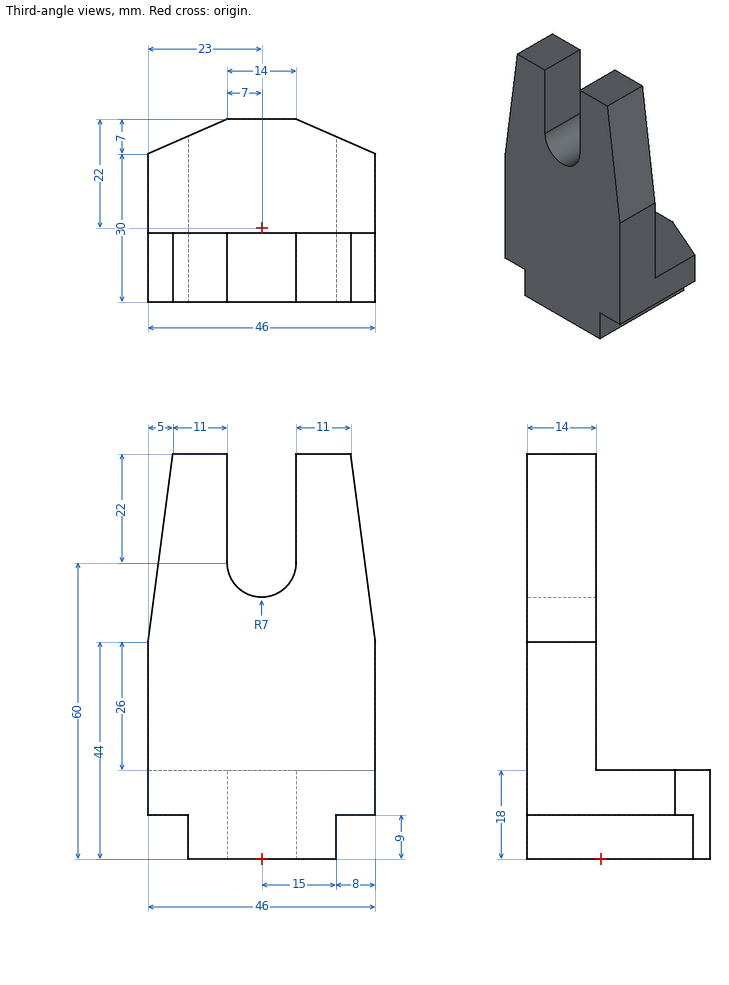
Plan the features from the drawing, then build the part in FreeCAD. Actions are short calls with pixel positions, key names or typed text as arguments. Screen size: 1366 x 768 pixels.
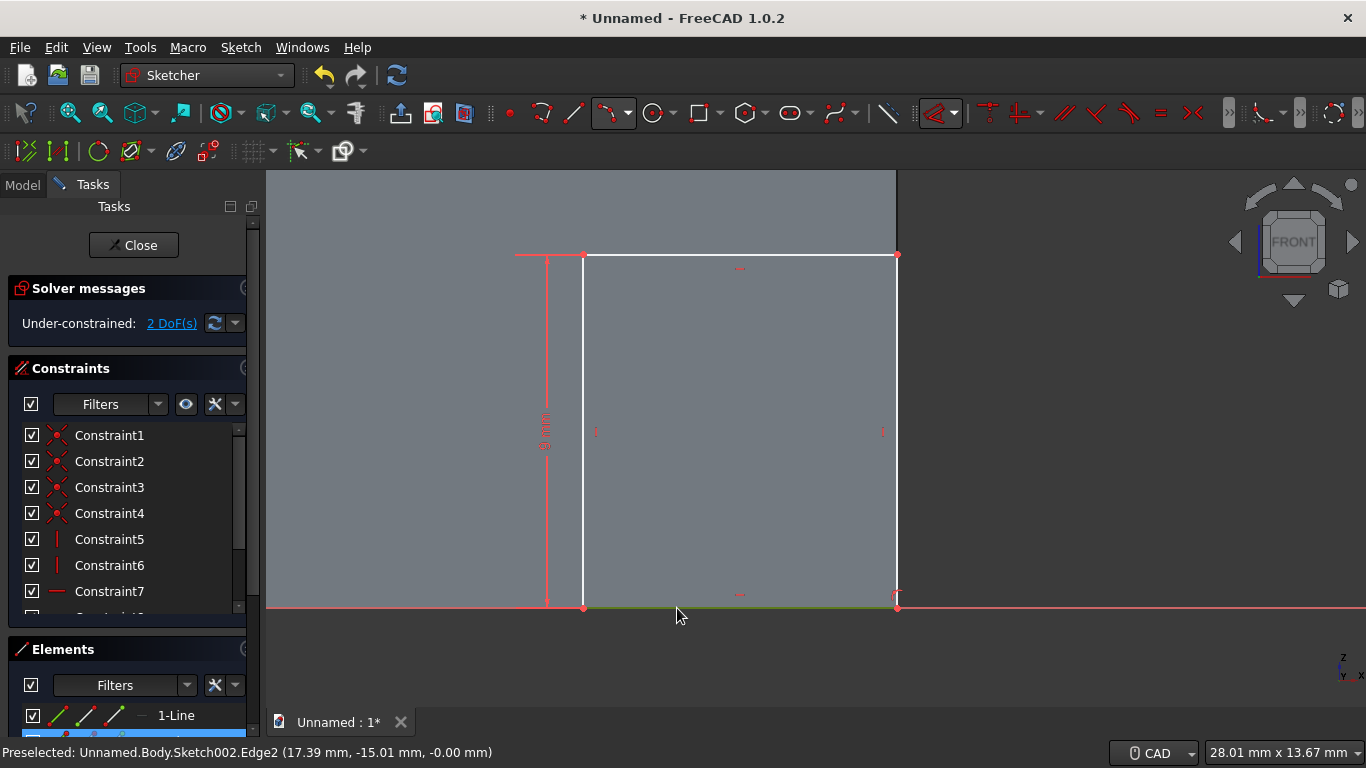
click(956, 114)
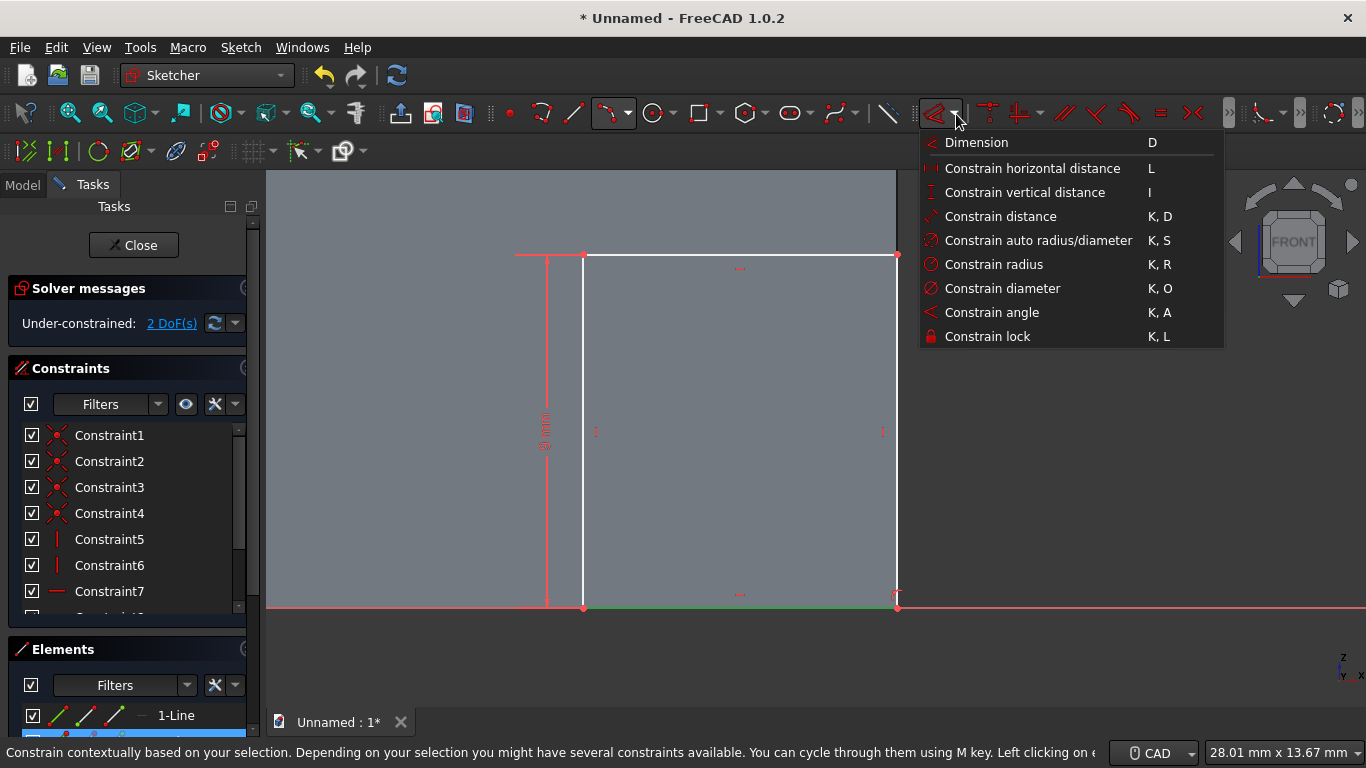
click(1072, 168)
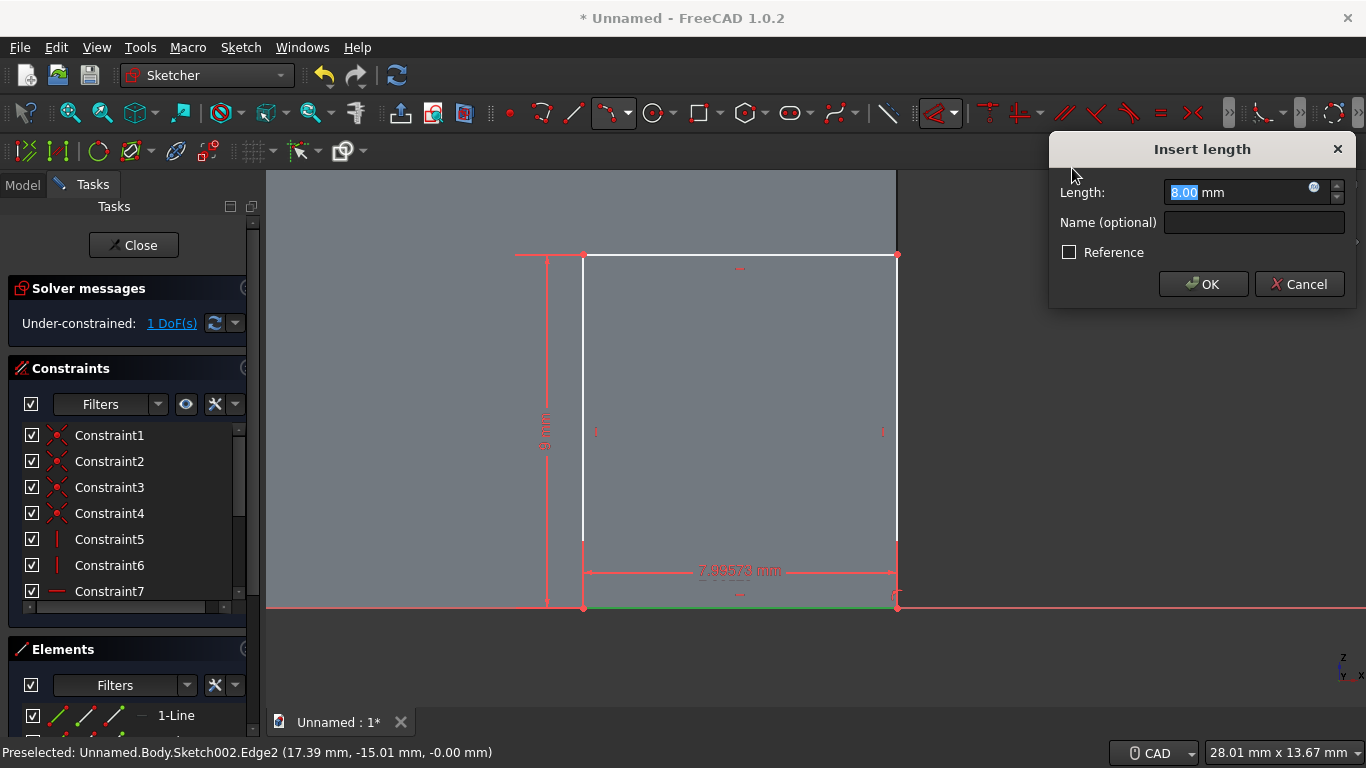
text(8)
key(Return)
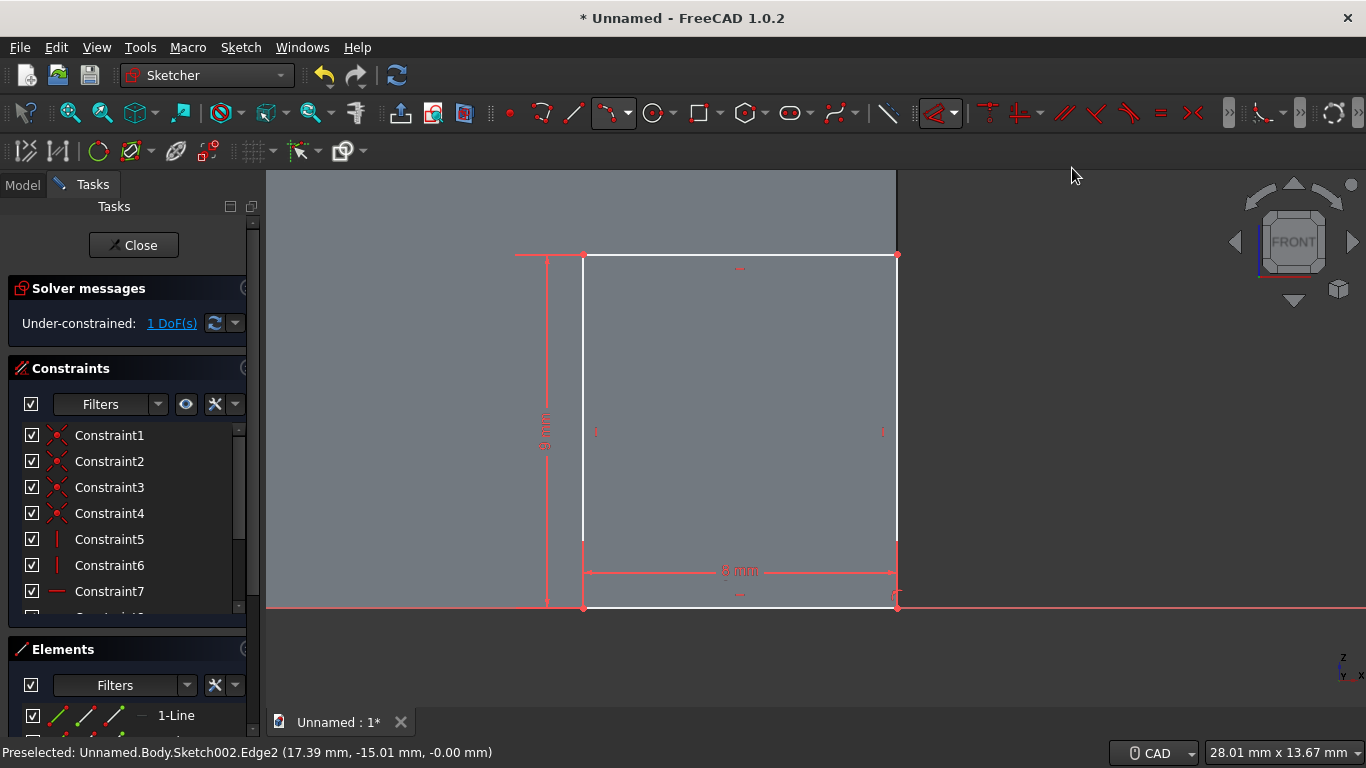
click(583, 255)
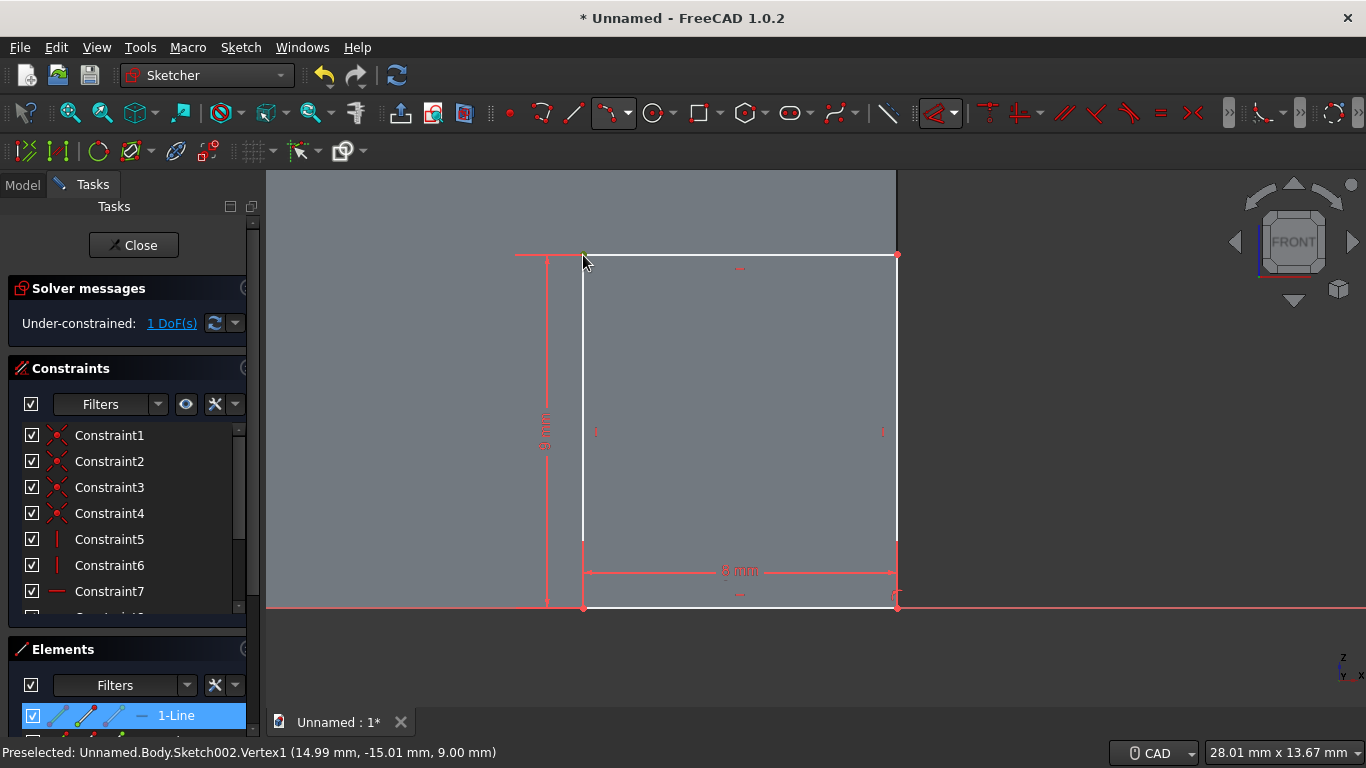
click(956, 114)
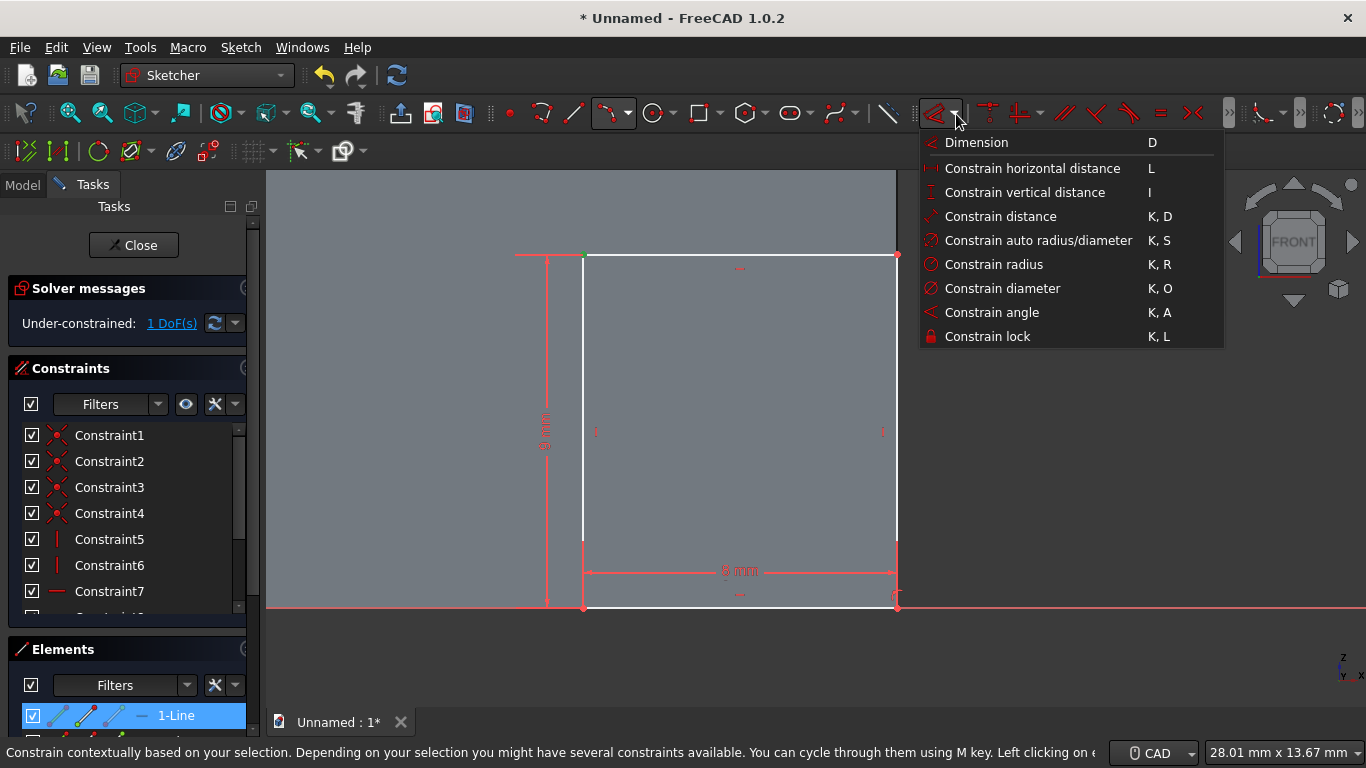
click(1072, 168)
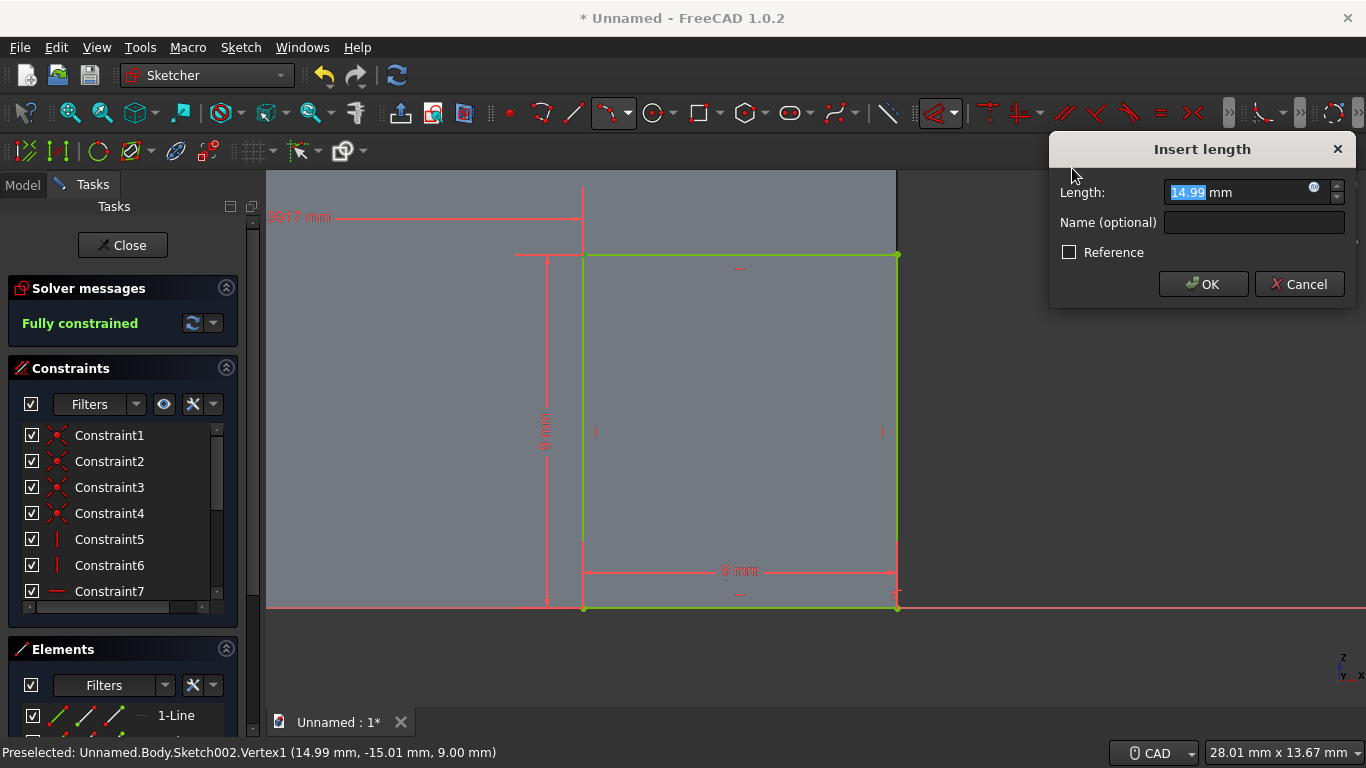
text(15)
key(Return)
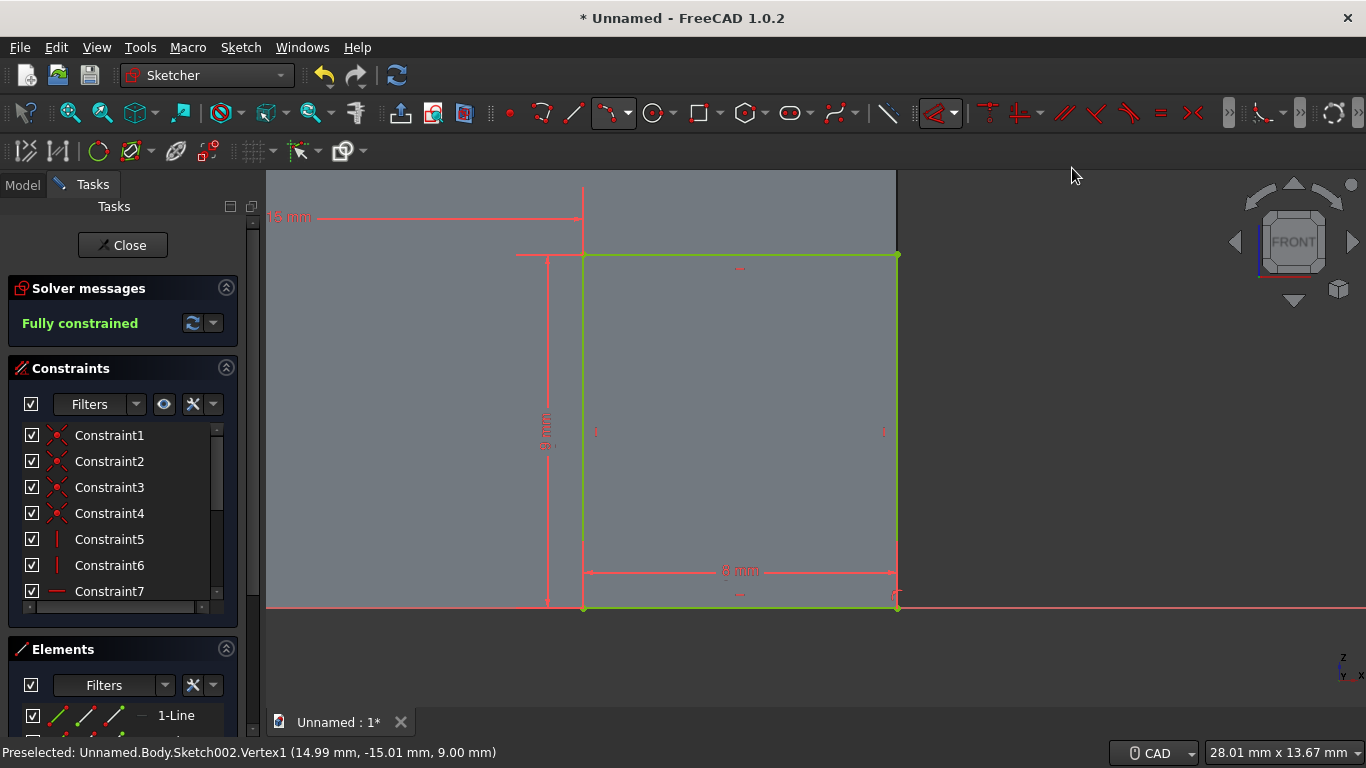
click(123, 245)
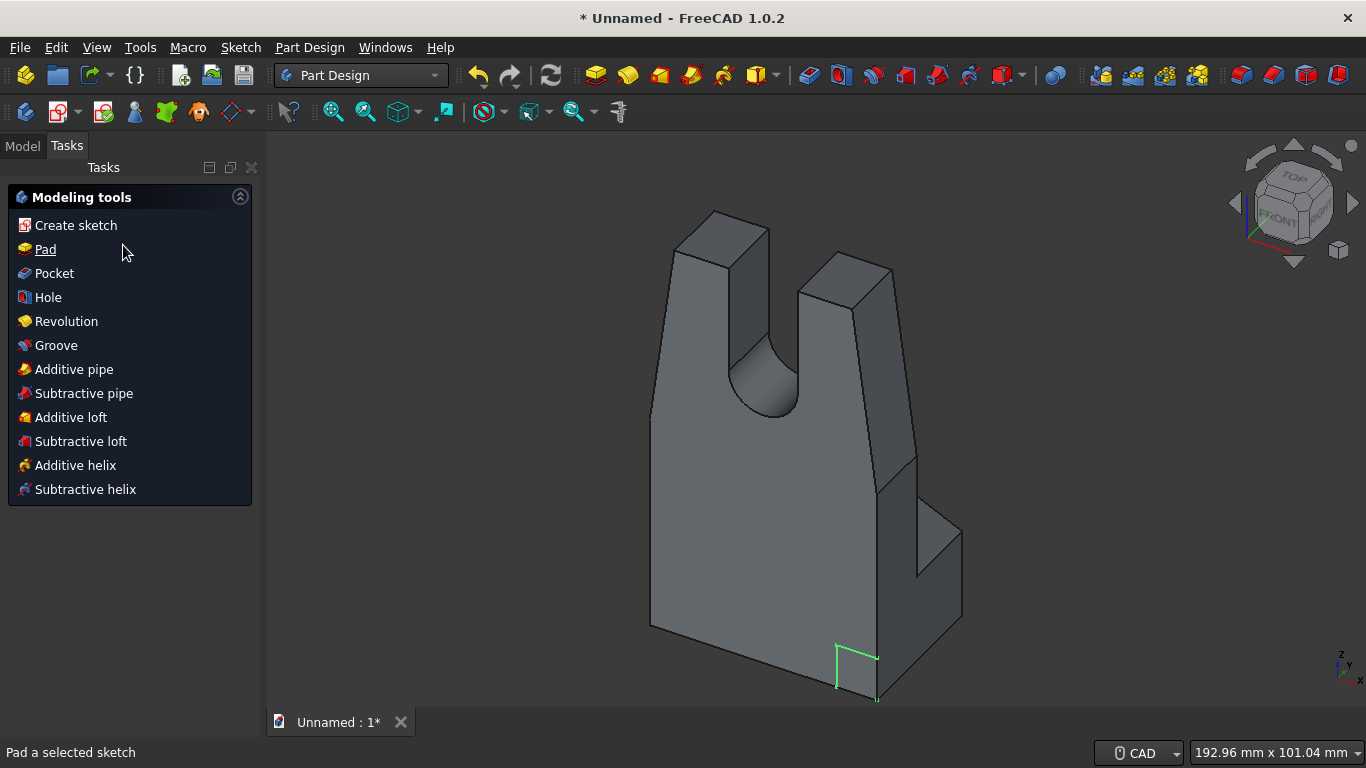
click(810, 76)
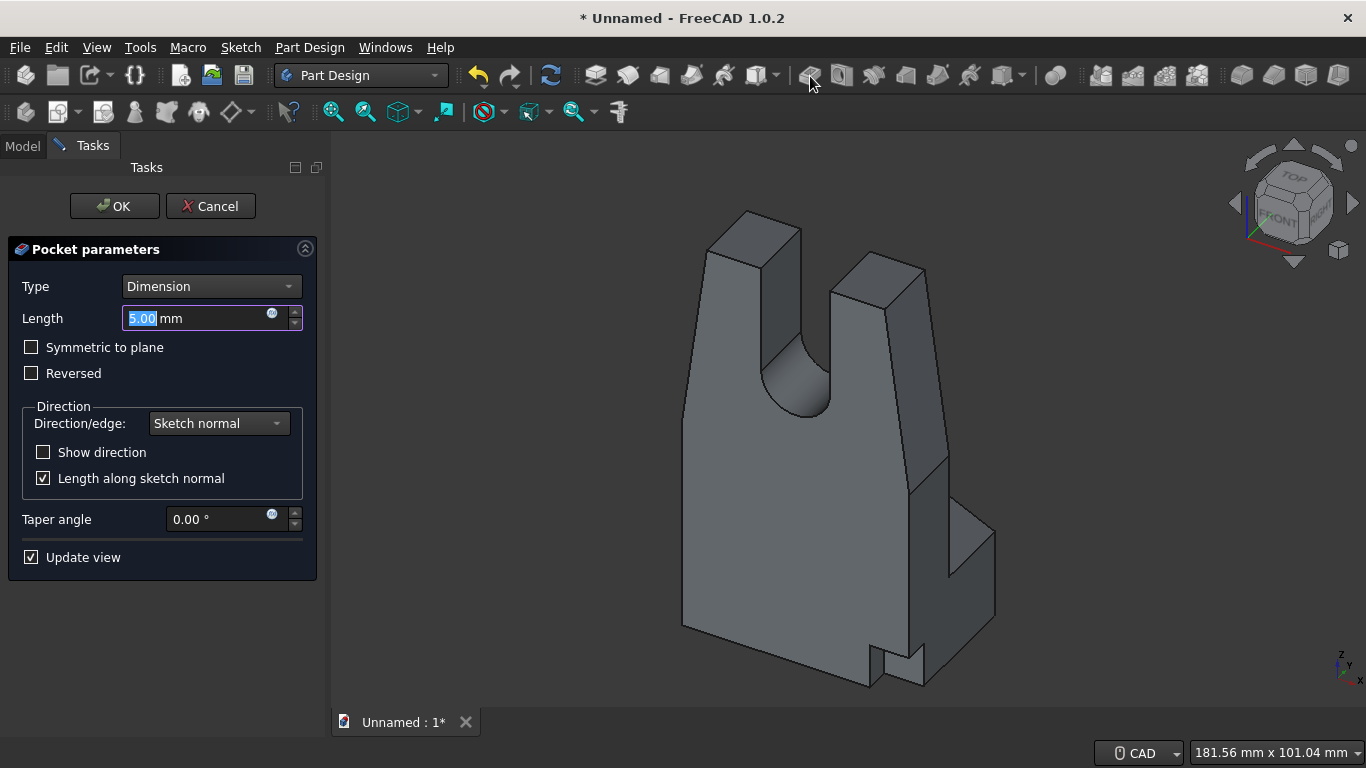
click(212, 286)